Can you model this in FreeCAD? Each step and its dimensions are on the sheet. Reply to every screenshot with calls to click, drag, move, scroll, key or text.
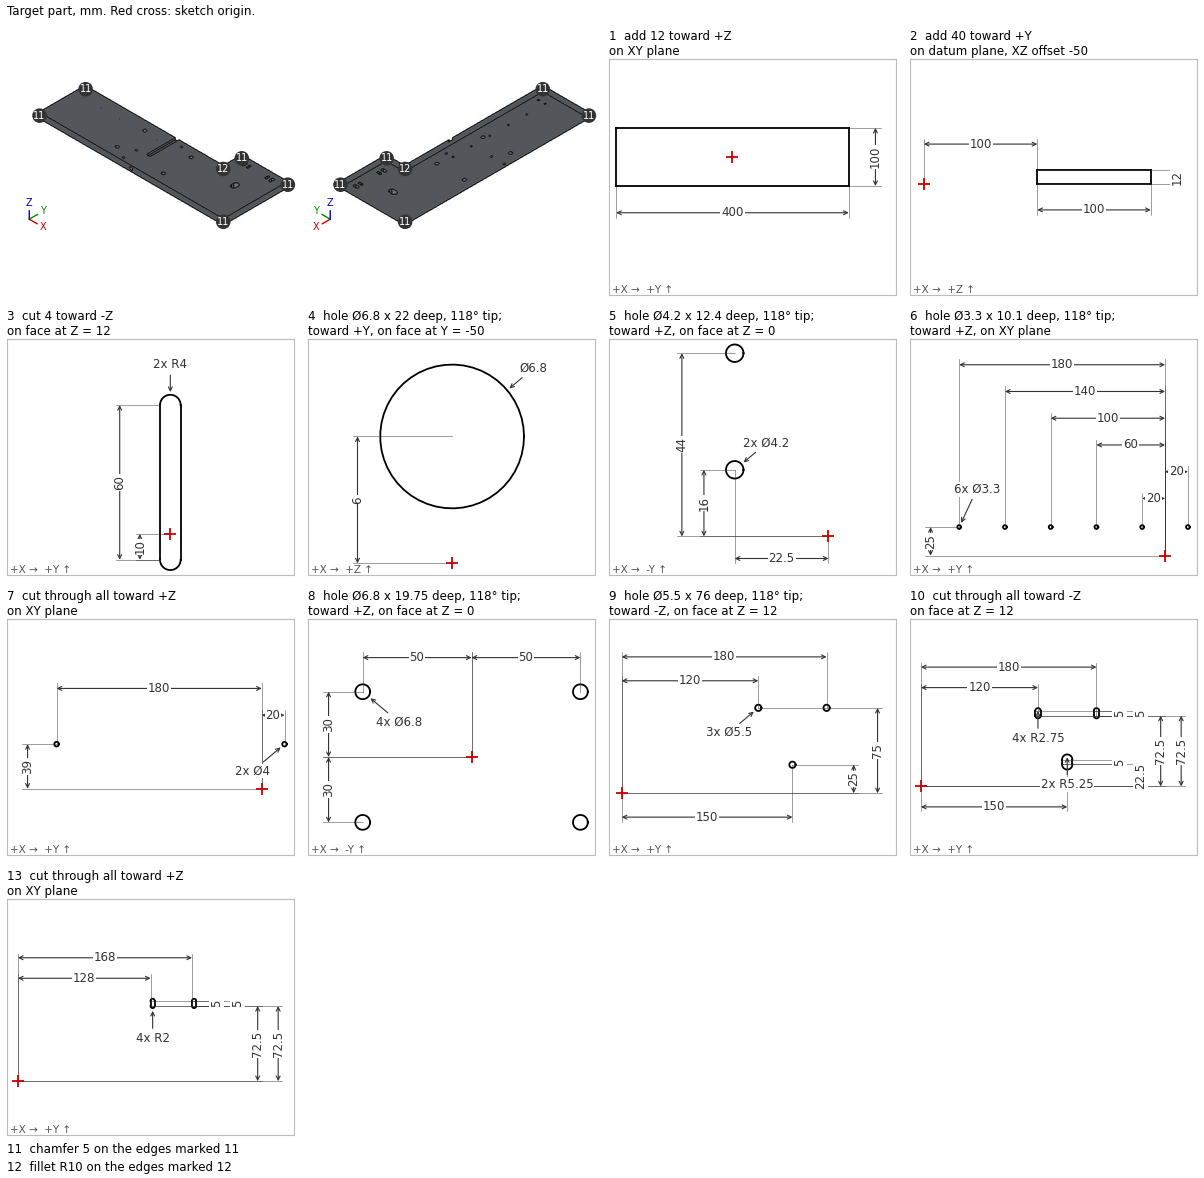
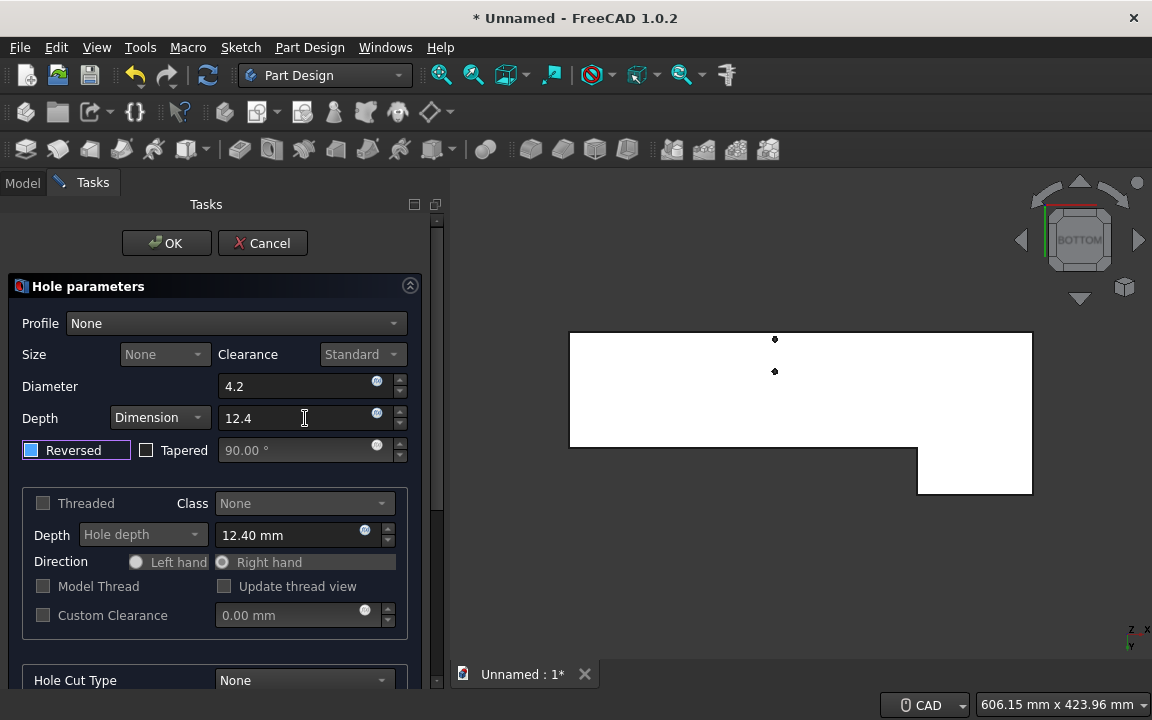
click(167, 243)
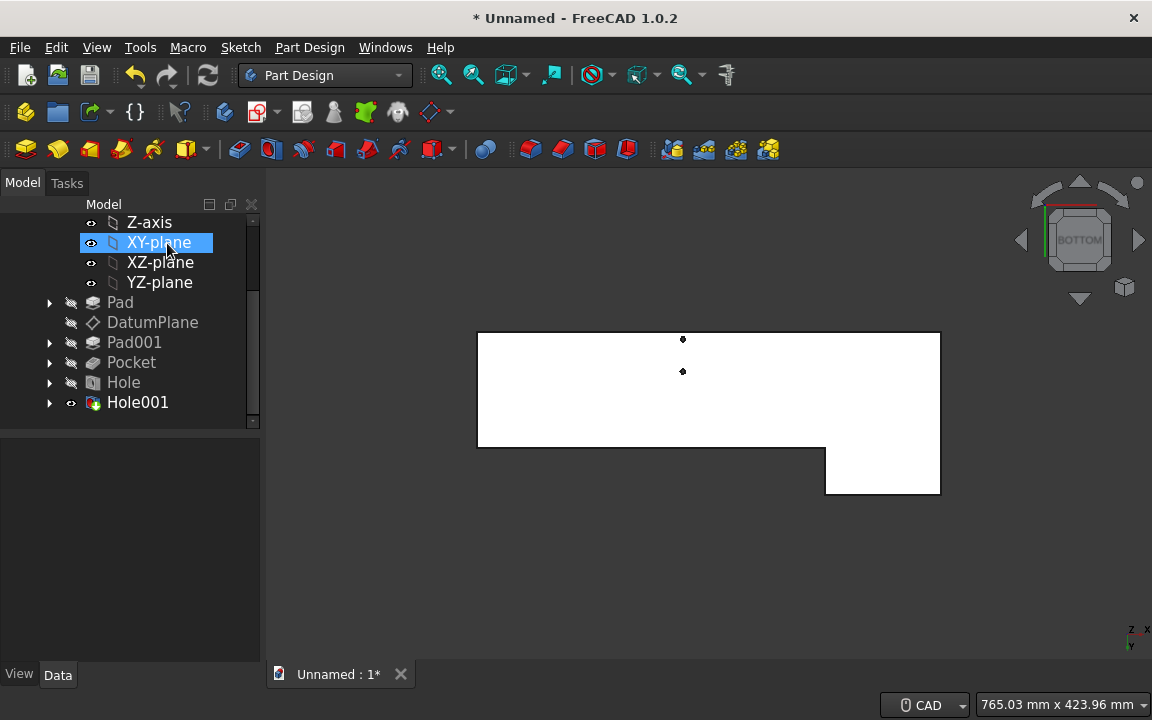
click(258, 112)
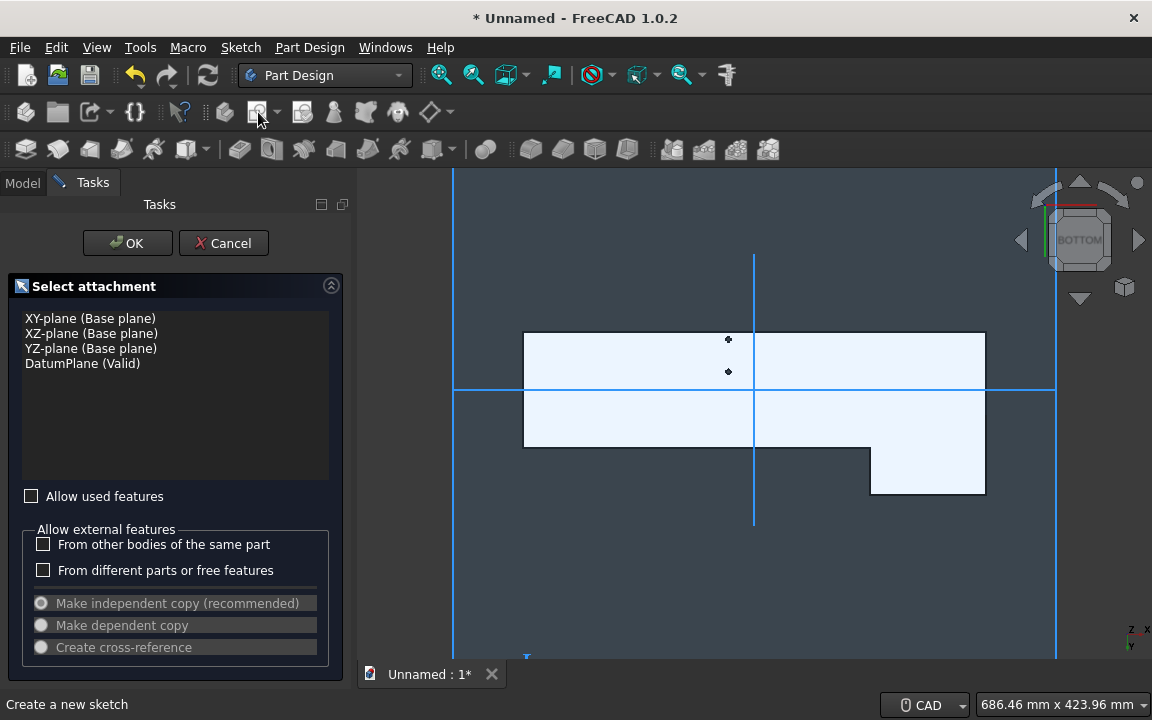
click(82, 318)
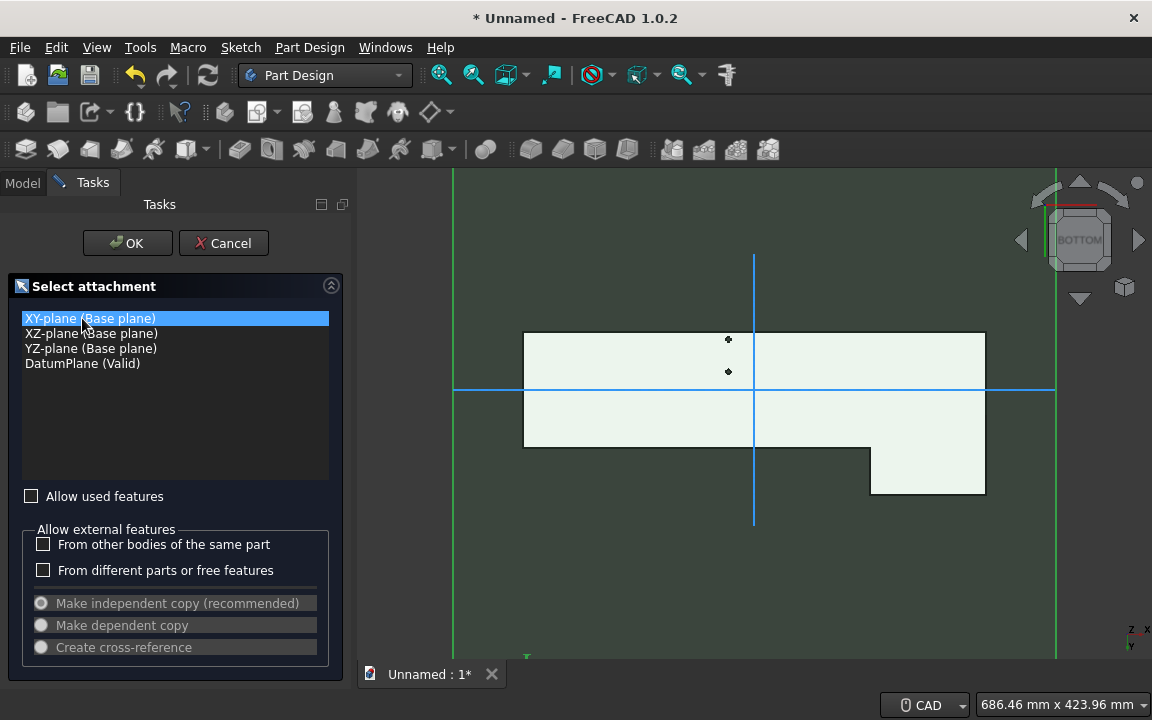
click(128, 243)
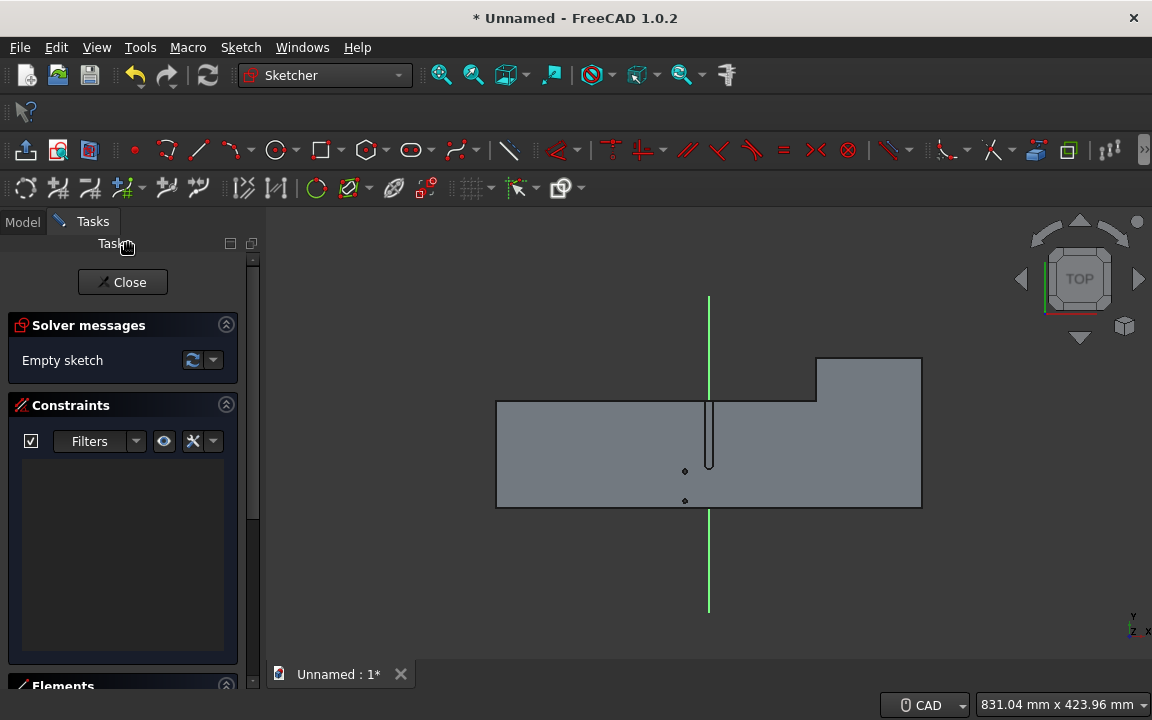
click(90, 150)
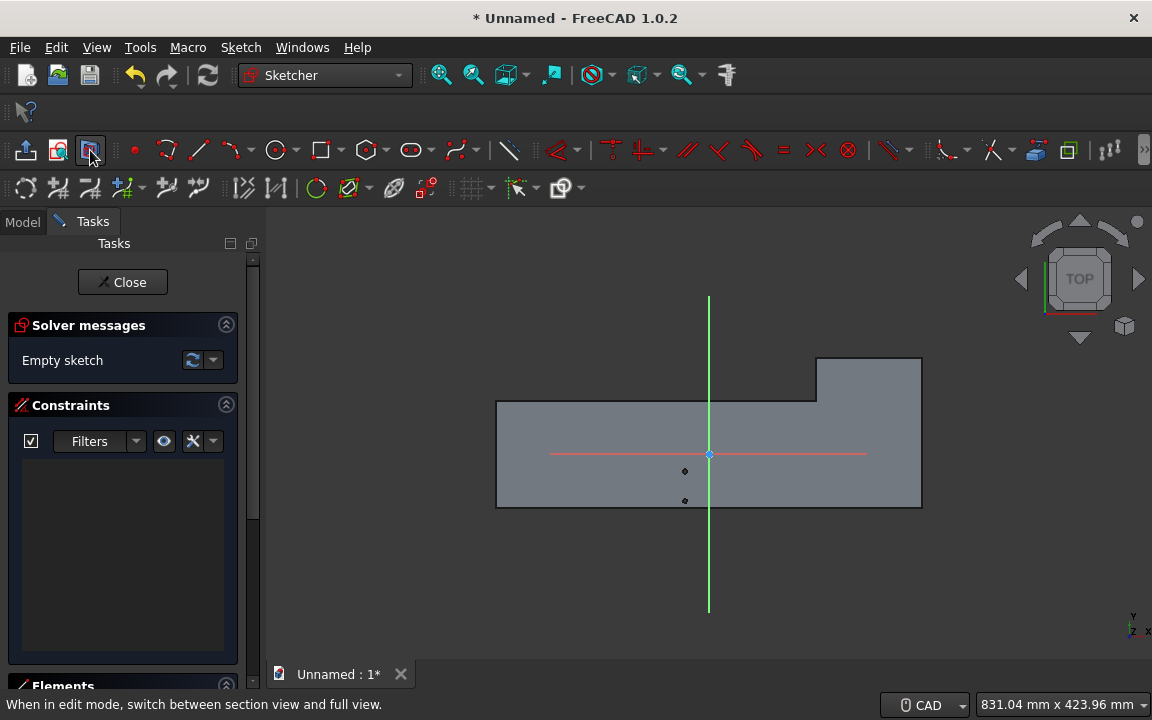
scroll(610, 446, up, 4)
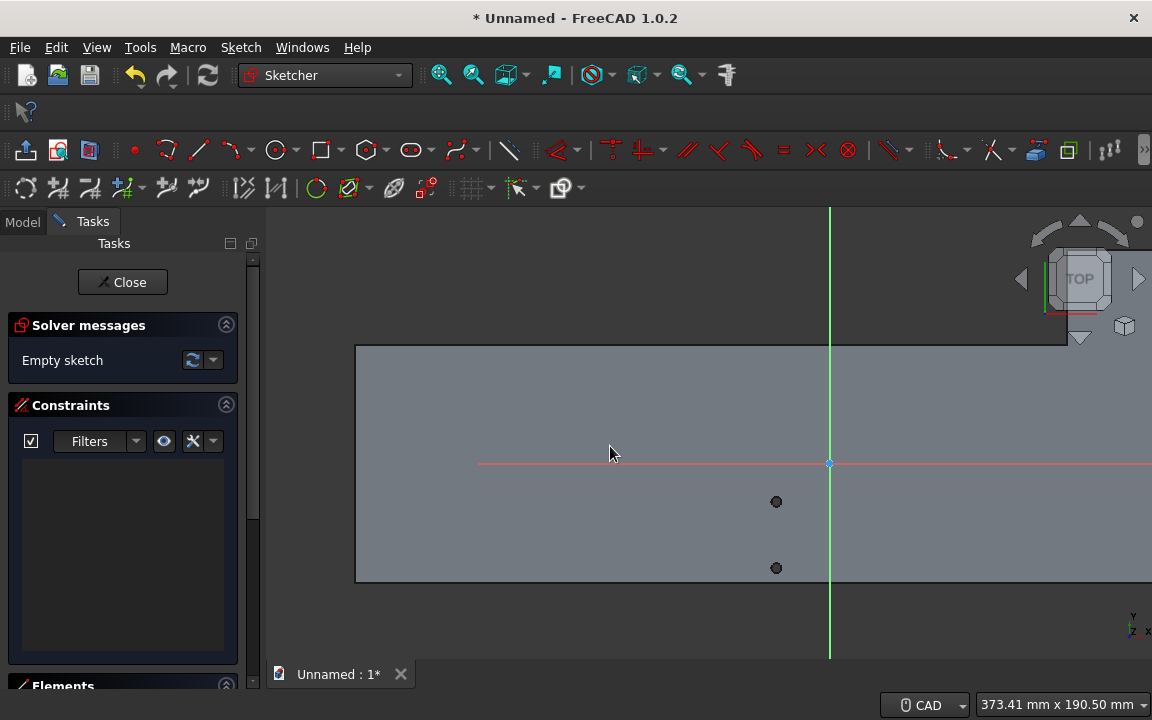
click(276, 150)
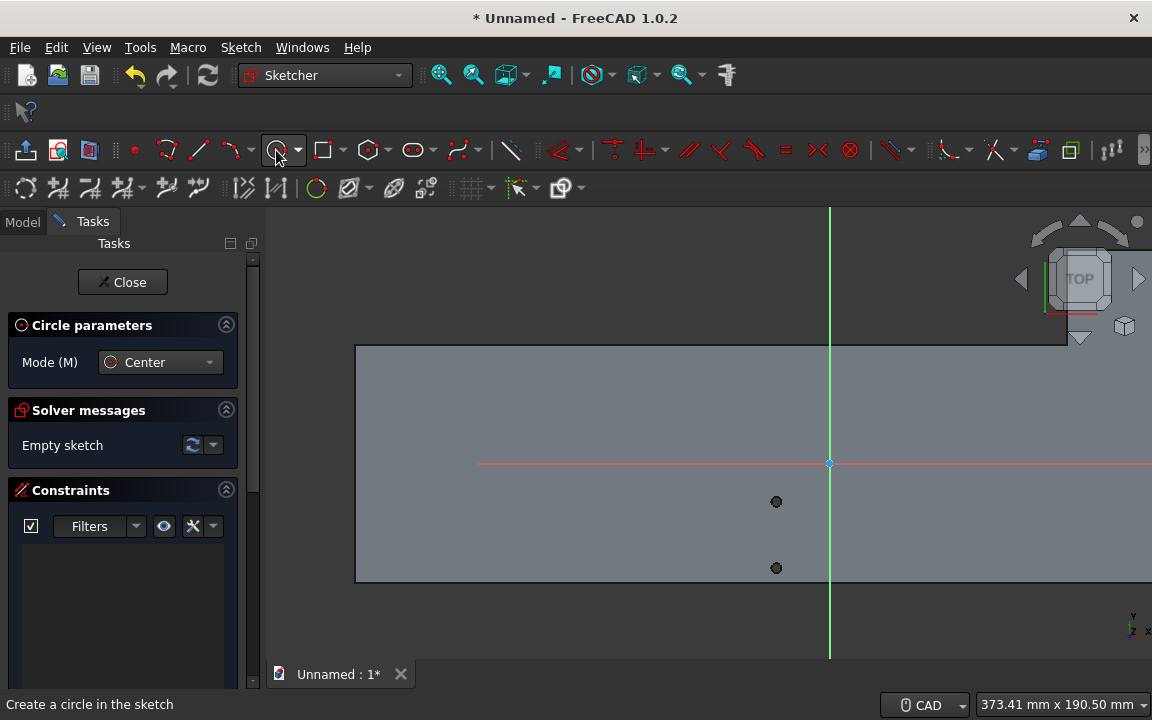
scroll(403, 405, up, 9)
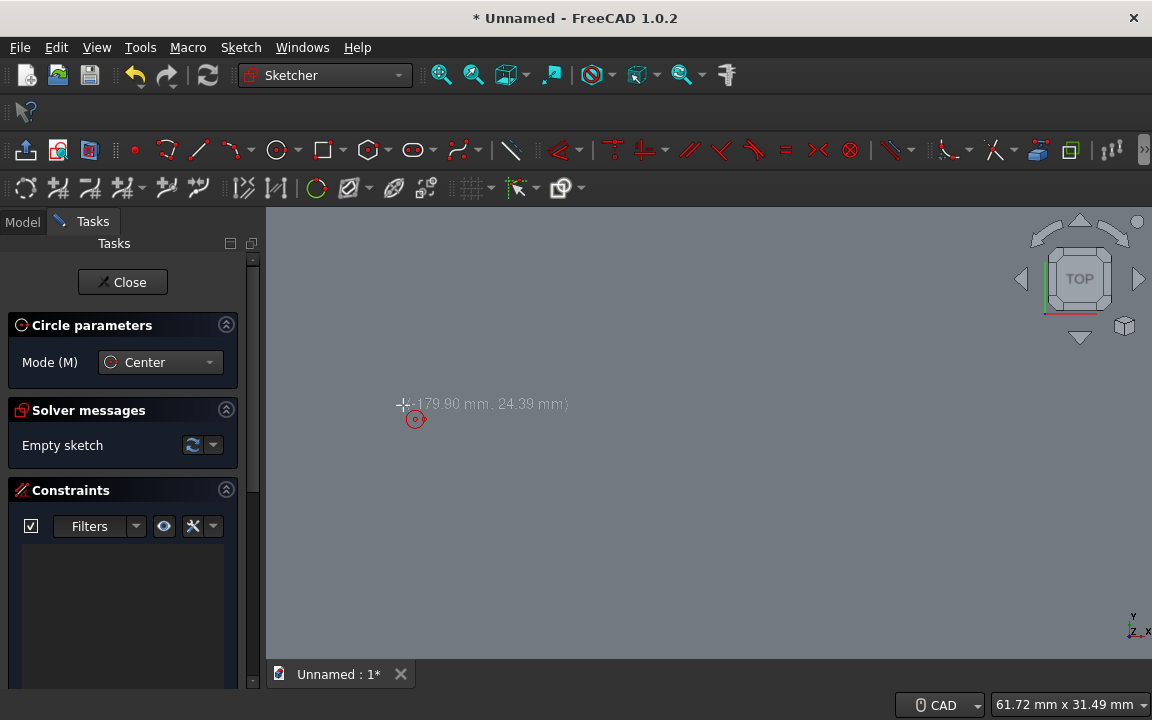
scroll(404, 406, down, 9)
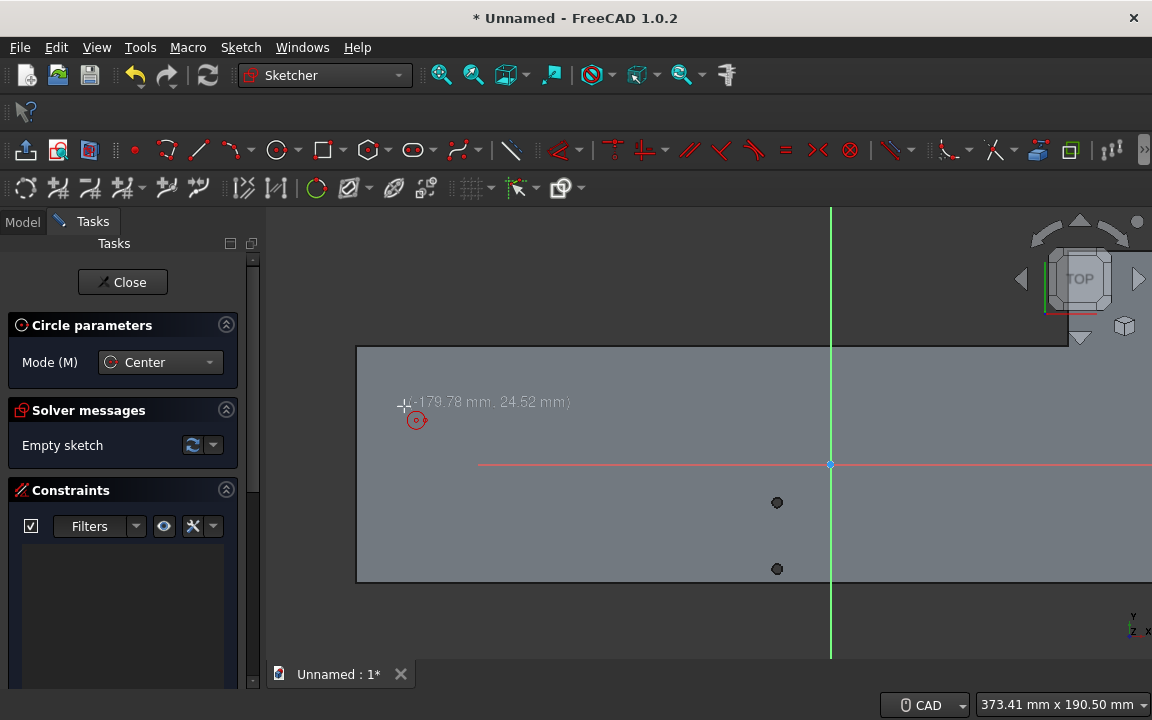
click(404, 405)
move(406, 403)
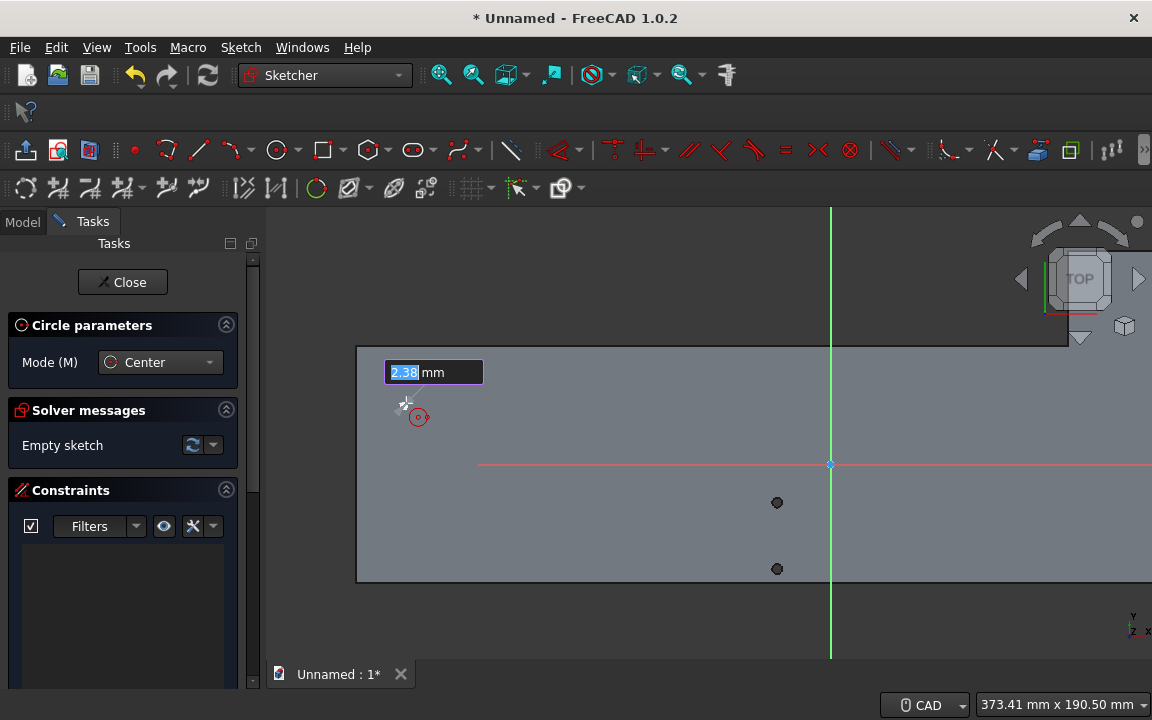
text(3.3)
key(Return)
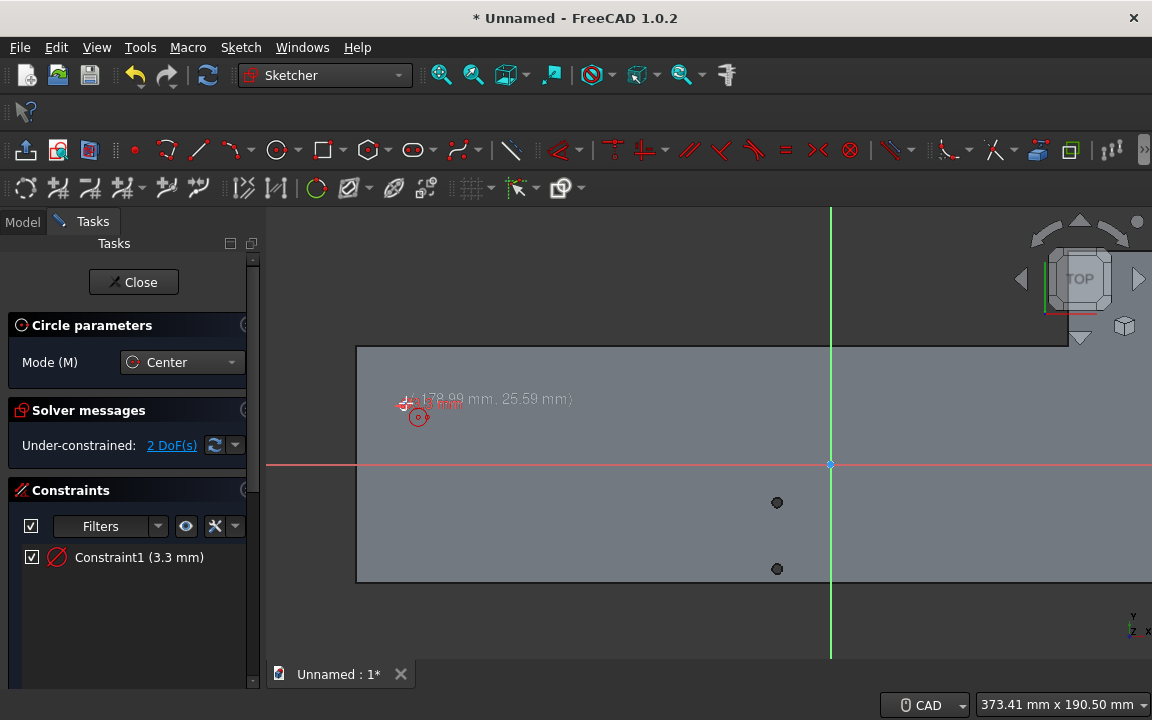
scroll(499, 405, up, 9)